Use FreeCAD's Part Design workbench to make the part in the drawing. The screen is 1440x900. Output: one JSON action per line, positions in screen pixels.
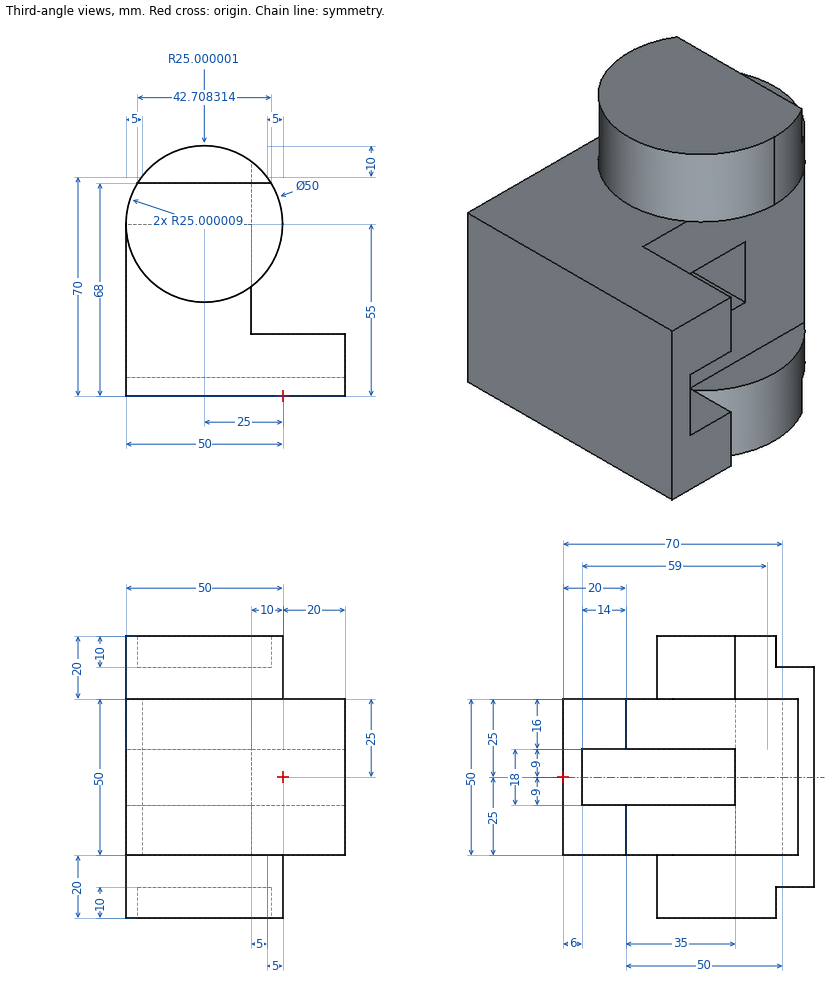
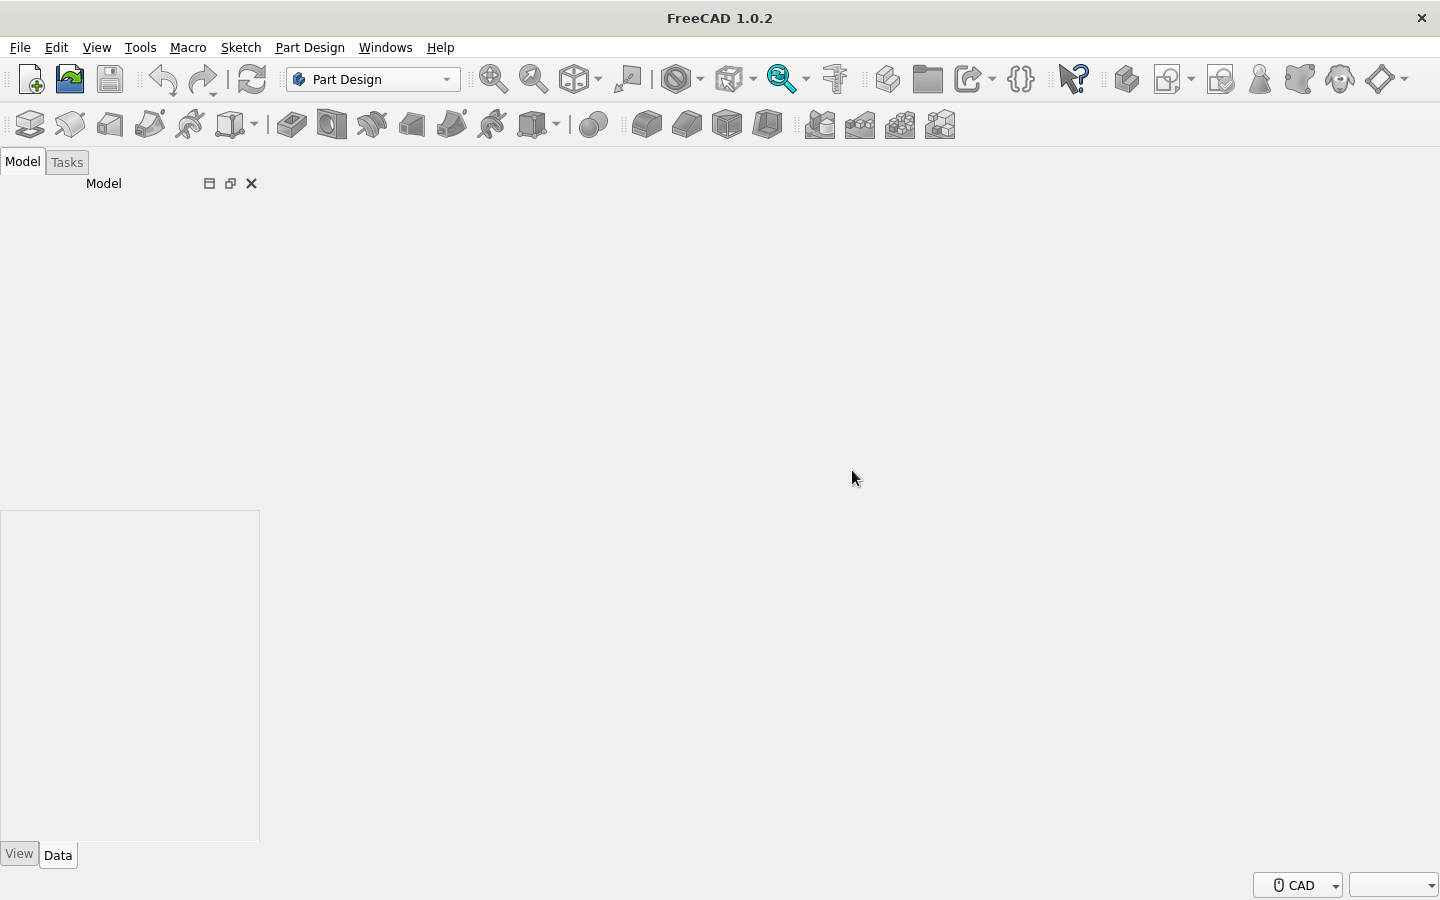
{"action": "left_click", "coordinate": [30, 80]}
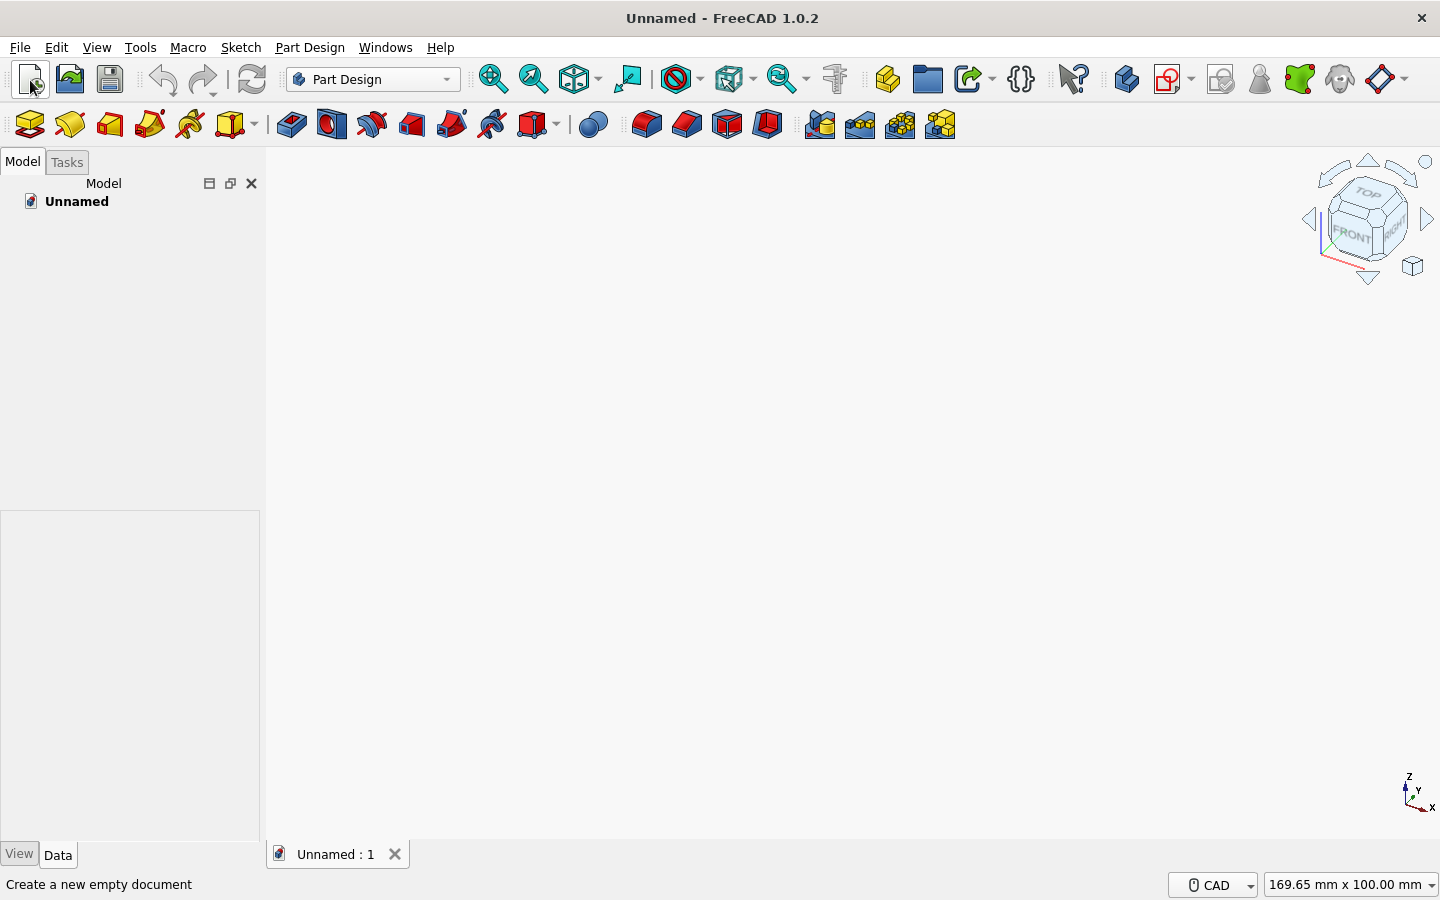
{"action": "left_click", "coordinate": [1168, 80]}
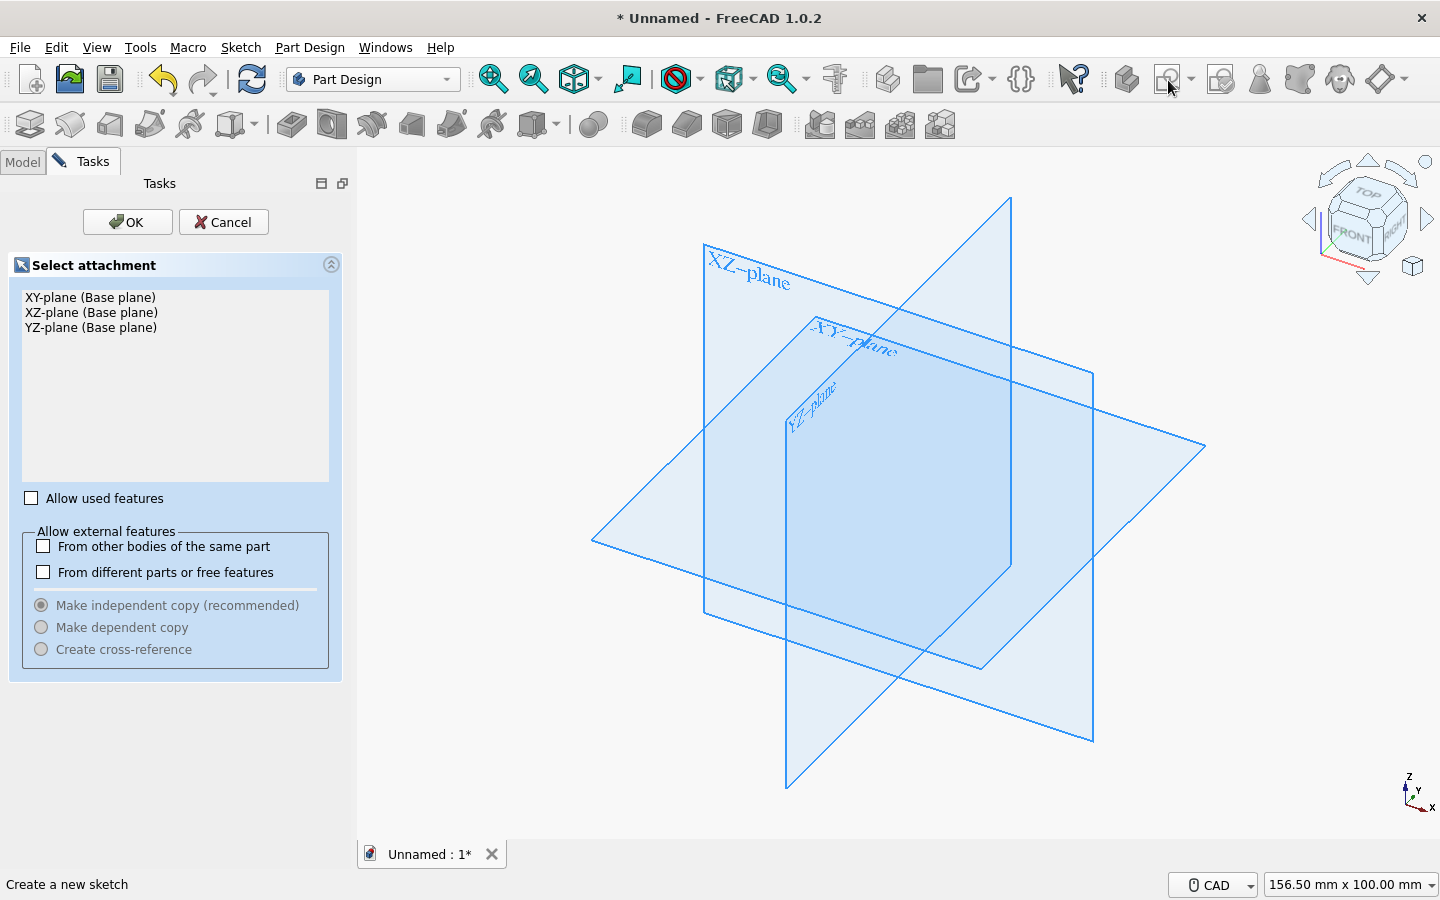
{"action": "left_click", "coordinate": [82, 328]}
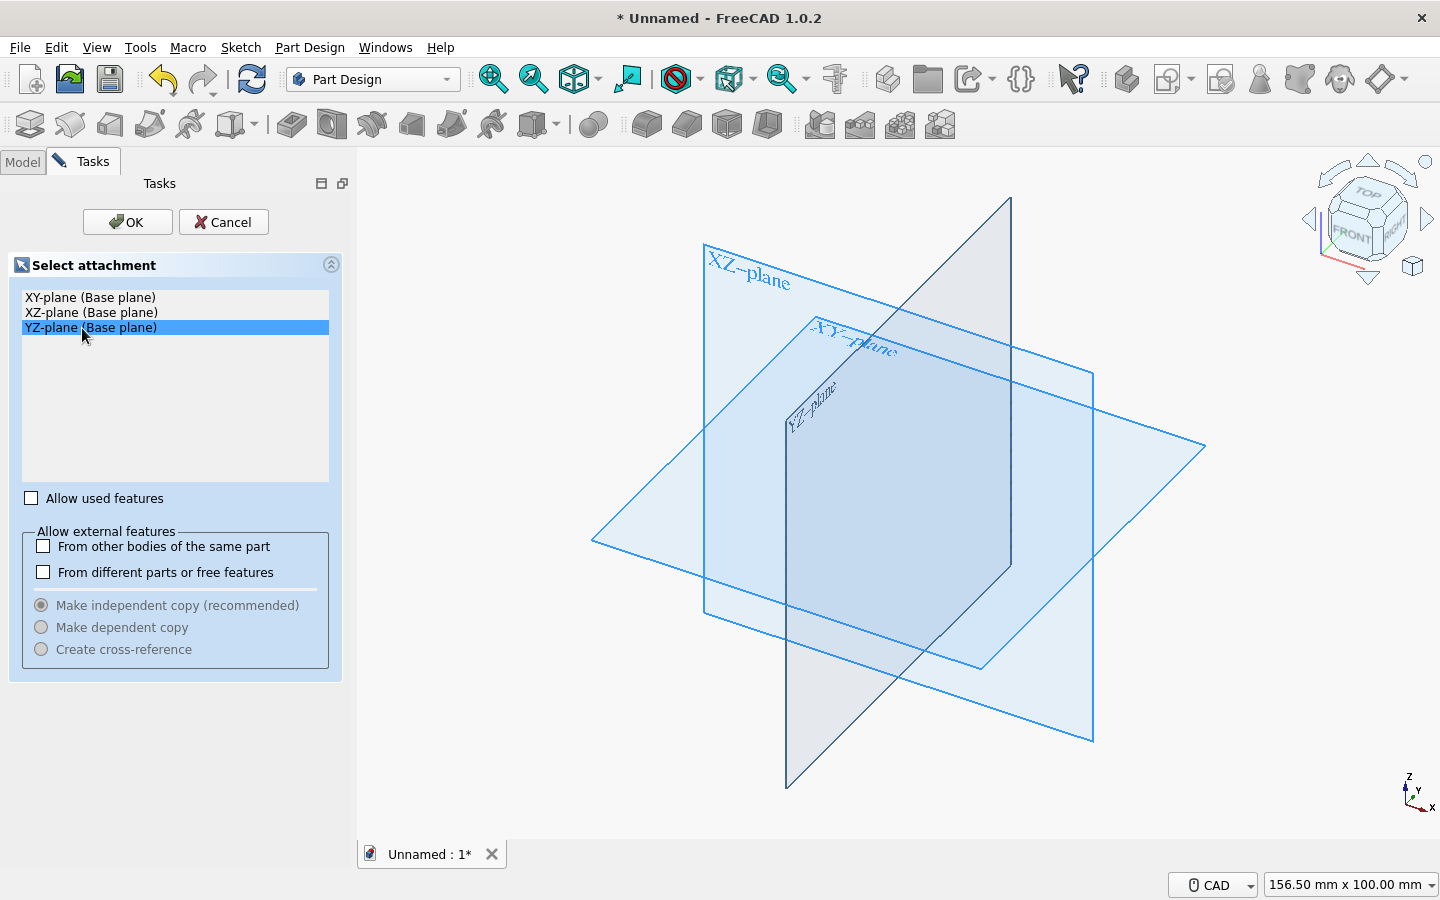
{"action": "left_click", "coordinate": [128, 222]}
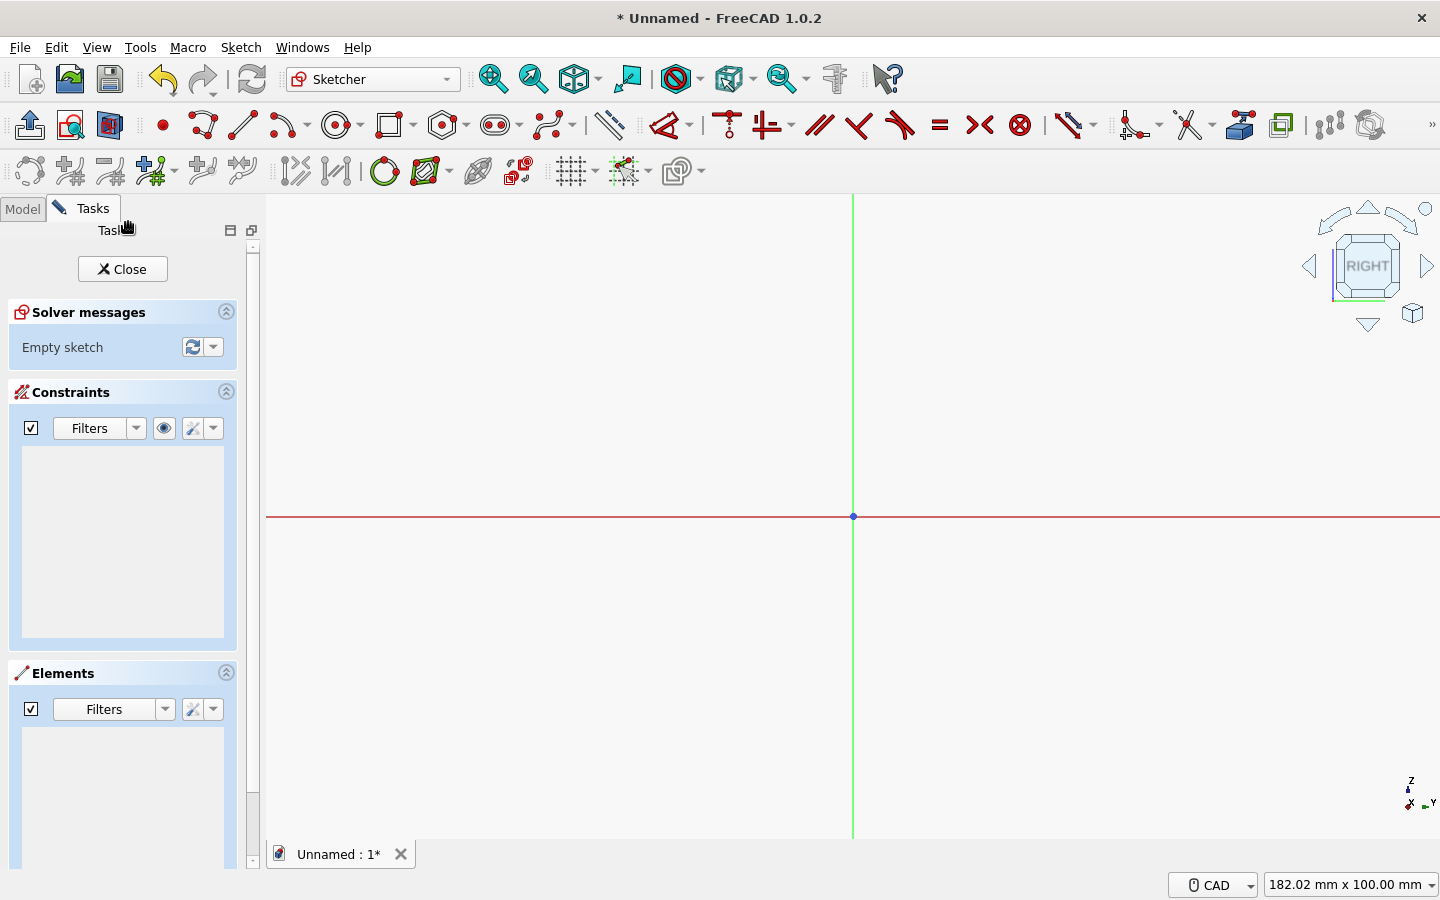
{"action": "left_click", "coordinate": [204, 126]}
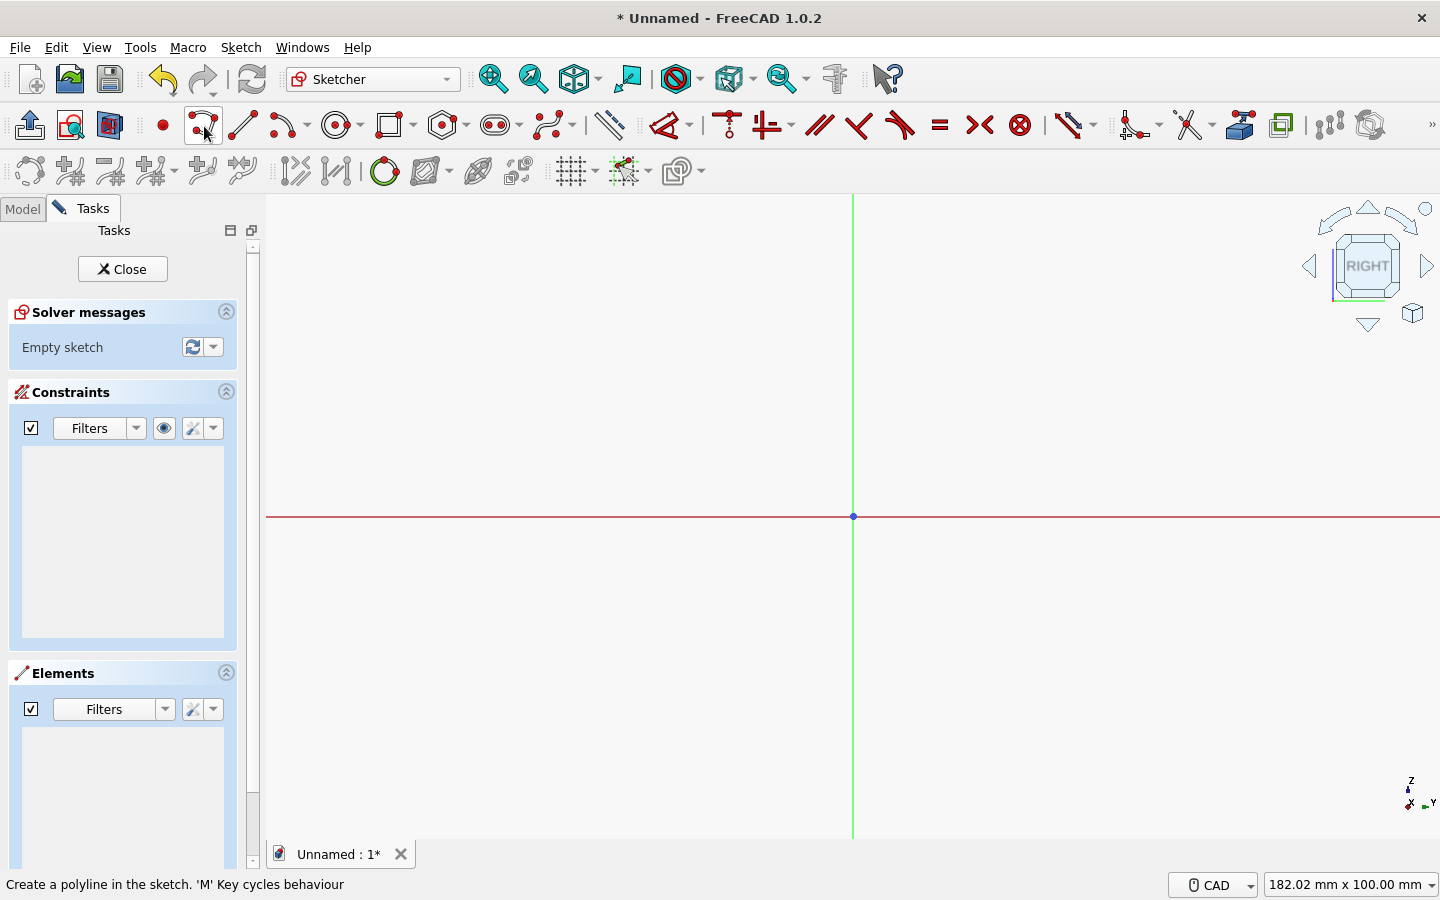
{"action": "left_click", "coordinate": [892, 575]}
{"action": "left_click", "coordinate": [892, 458]}
{"action": "left_click", "coordinate": [982, 458]}
{"action": "left_click", "coordinate": [982, 355]}
{"action": "left_click", "coordinate": [853, 355]}
{"action": "left_click", "coordinate": [862, 678]}
{"action": "left_click", "coordinate": [982, 678]}
{"action": "left_click", "coordinate": [982, 575]}
{"action": "left_click", "coordinate": [892, 576]}
{"action": "key", "text": "Escape"}
{"action": "key", "text": "Escape"}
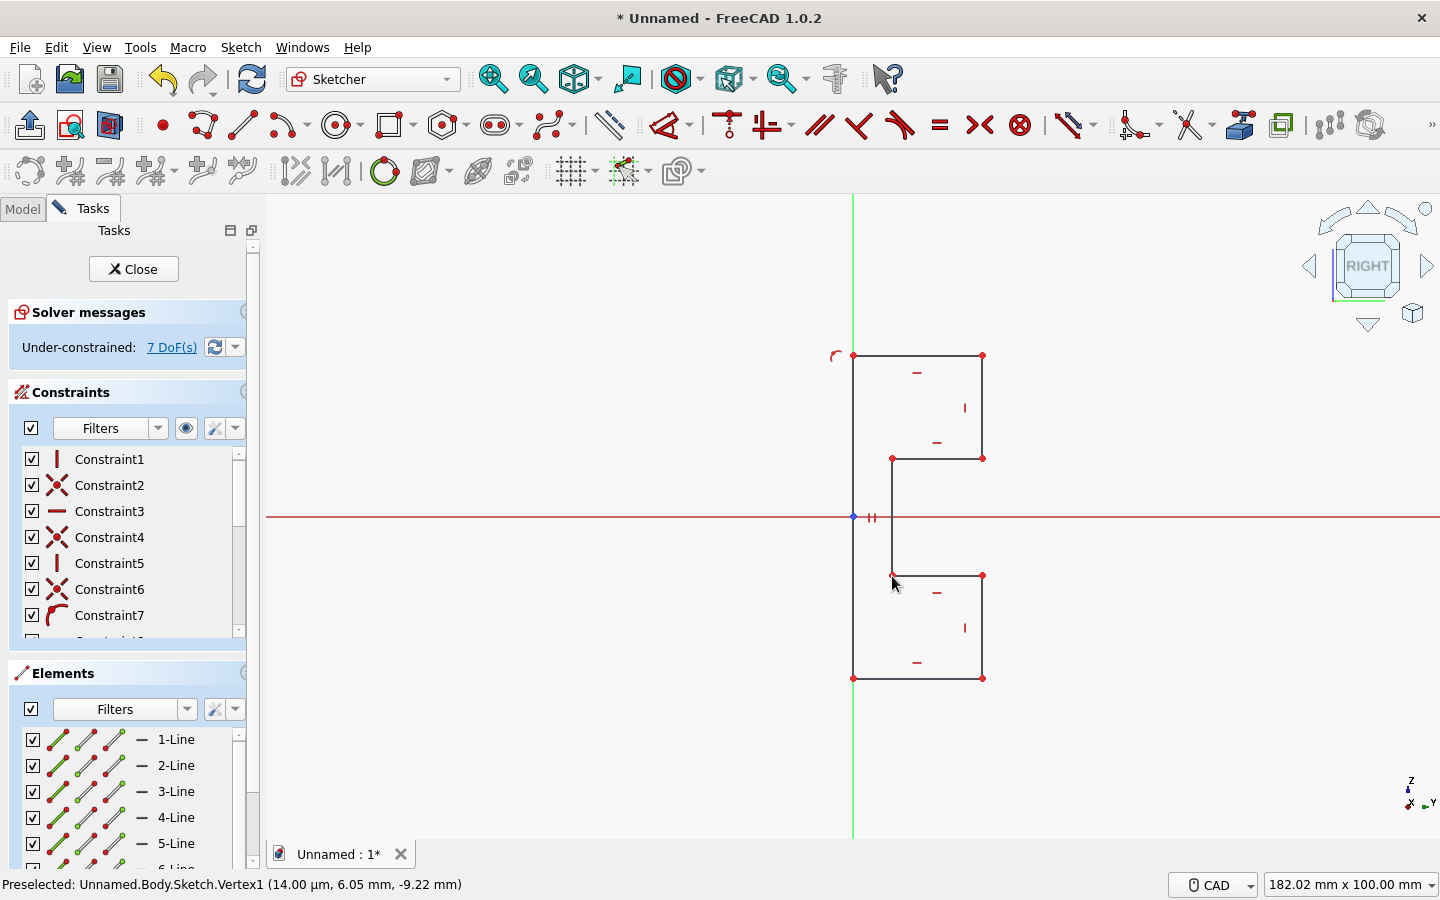
{"action": "left_click", "coordinate": [982, 356]}